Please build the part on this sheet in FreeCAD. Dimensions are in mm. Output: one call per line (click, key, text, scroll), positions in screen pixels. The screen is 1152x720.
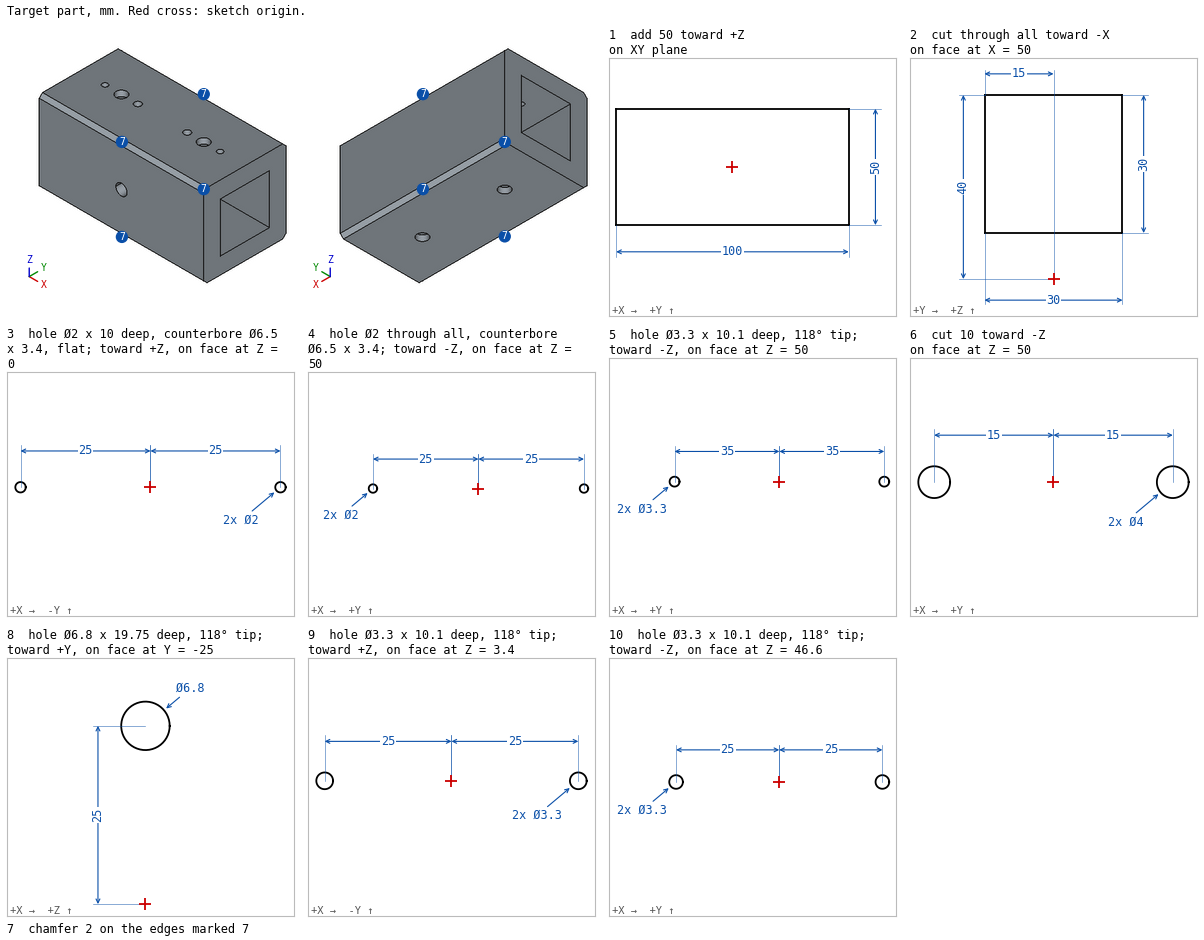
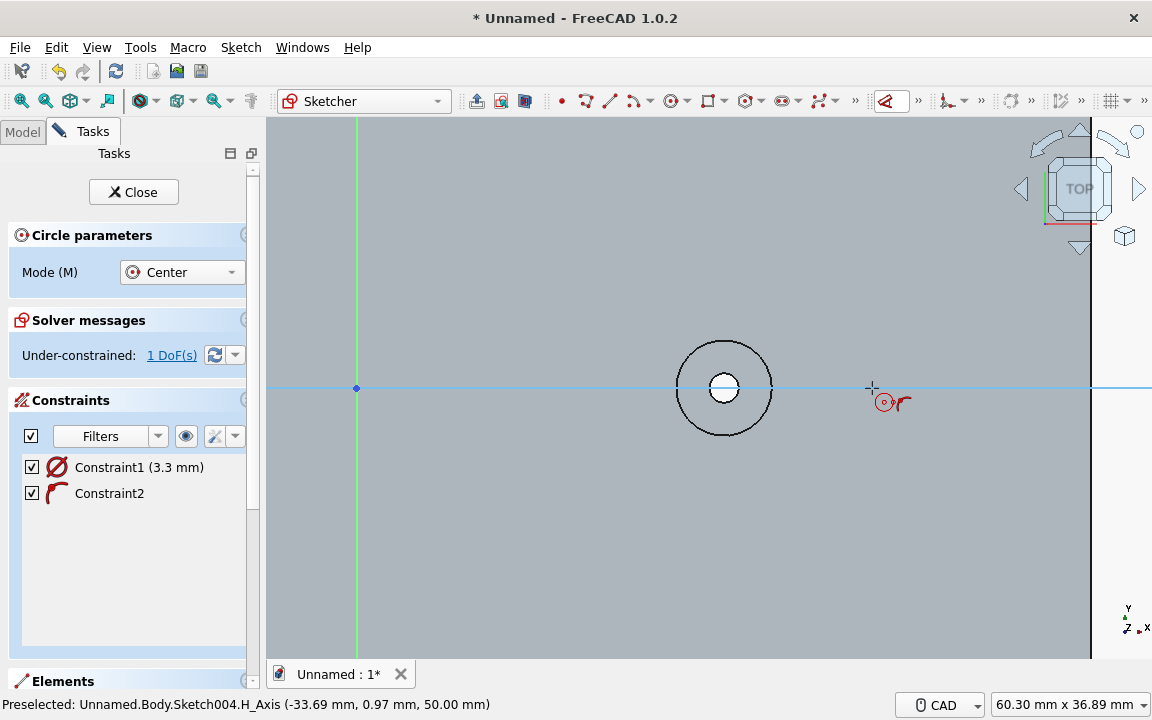
click(871, 388)
move(888, 371)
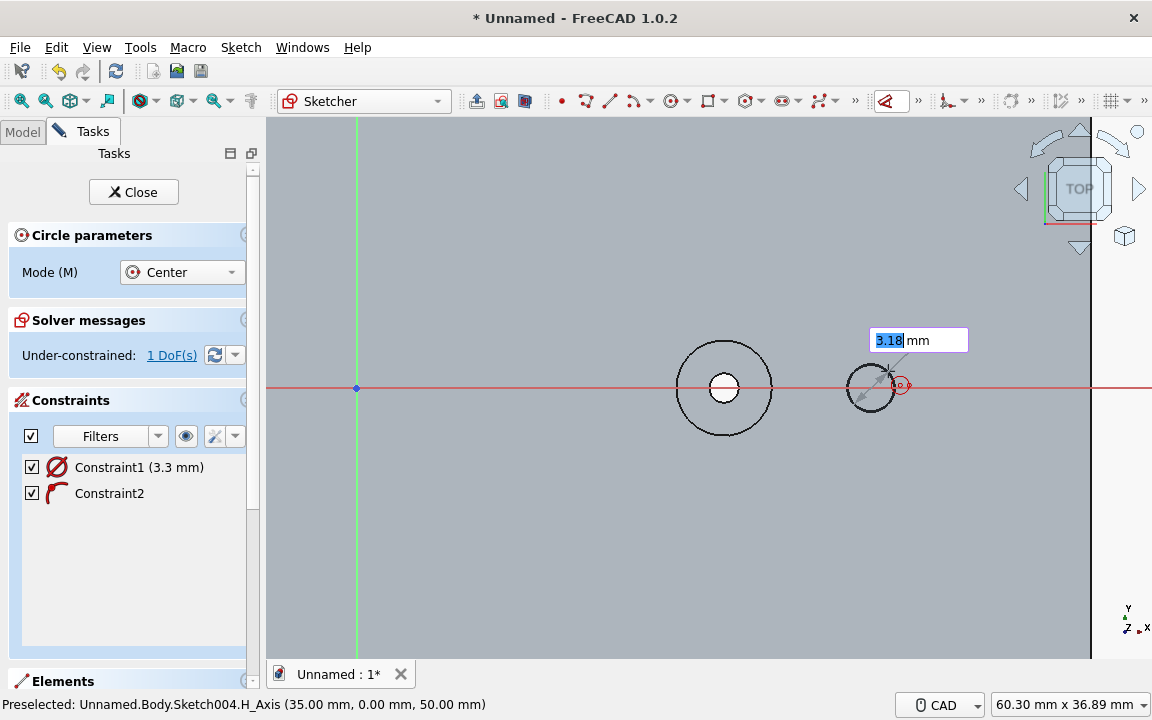
text(3.3)
key(Return)
key(Escape)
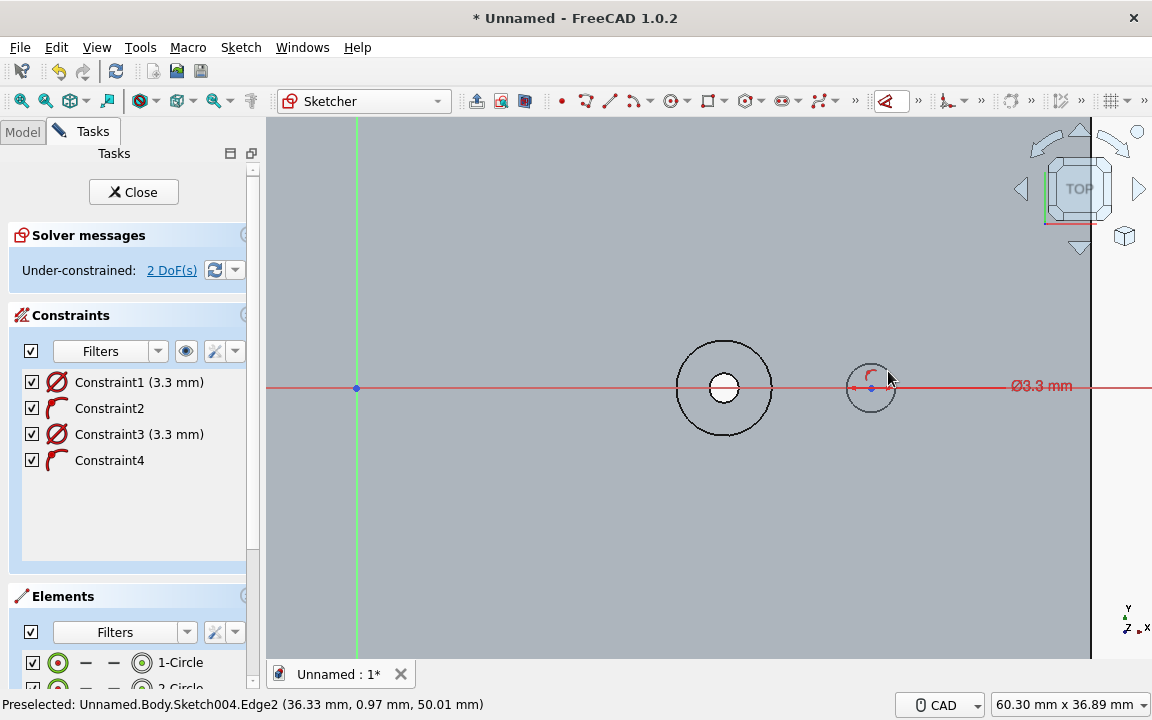
scroll(872, 388, down, 4)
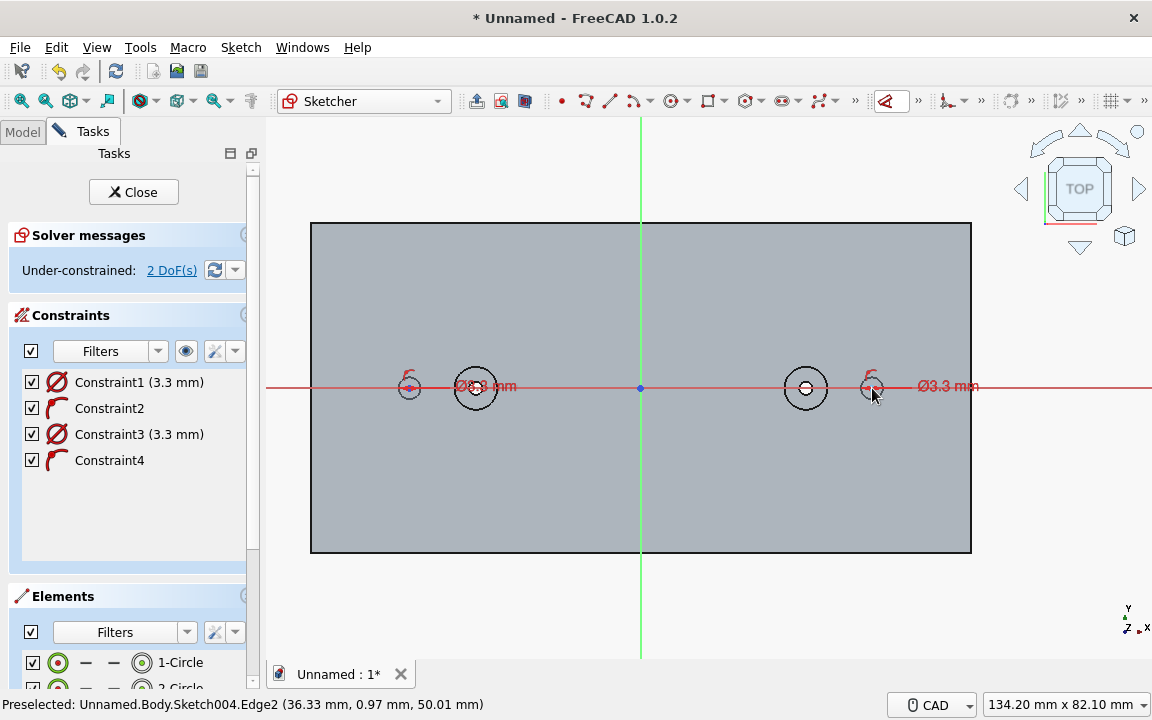
click(410, 388)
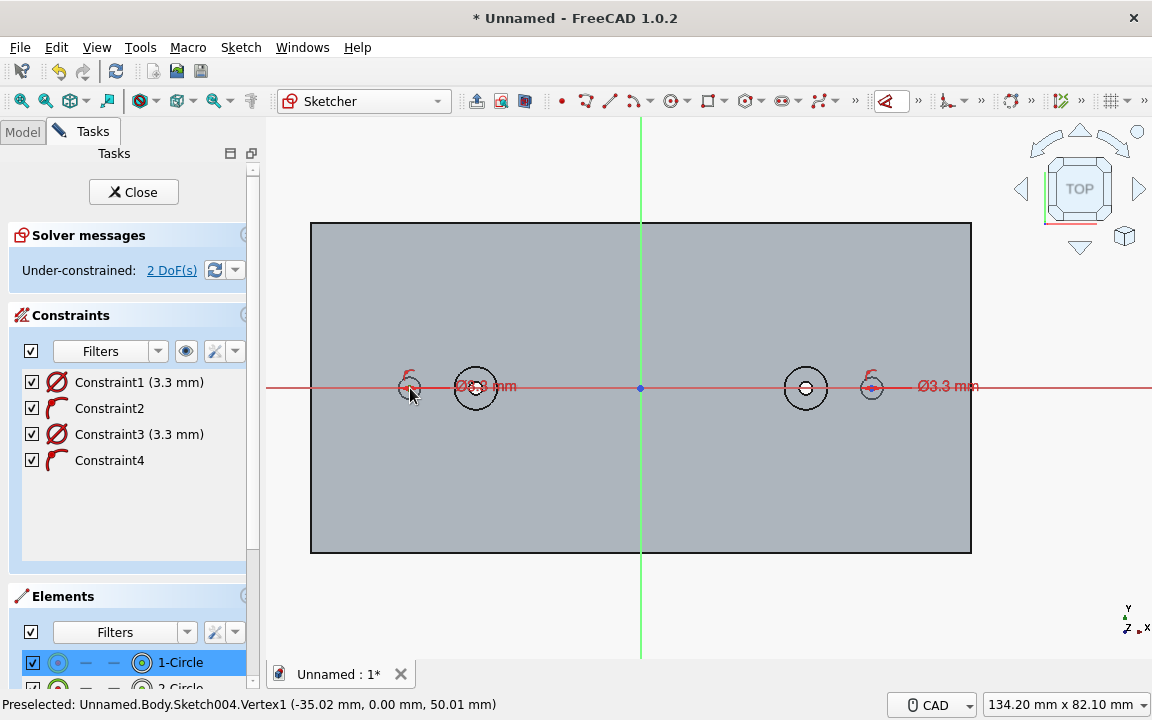
key(l)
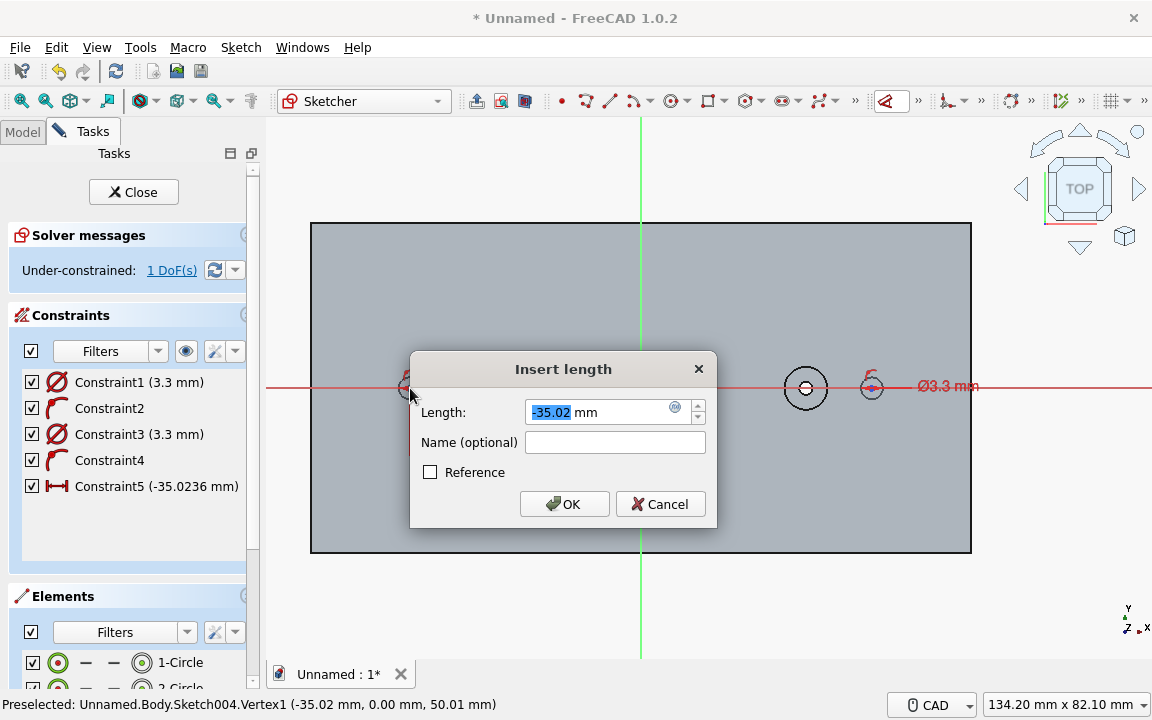
text(-35)
key(Return)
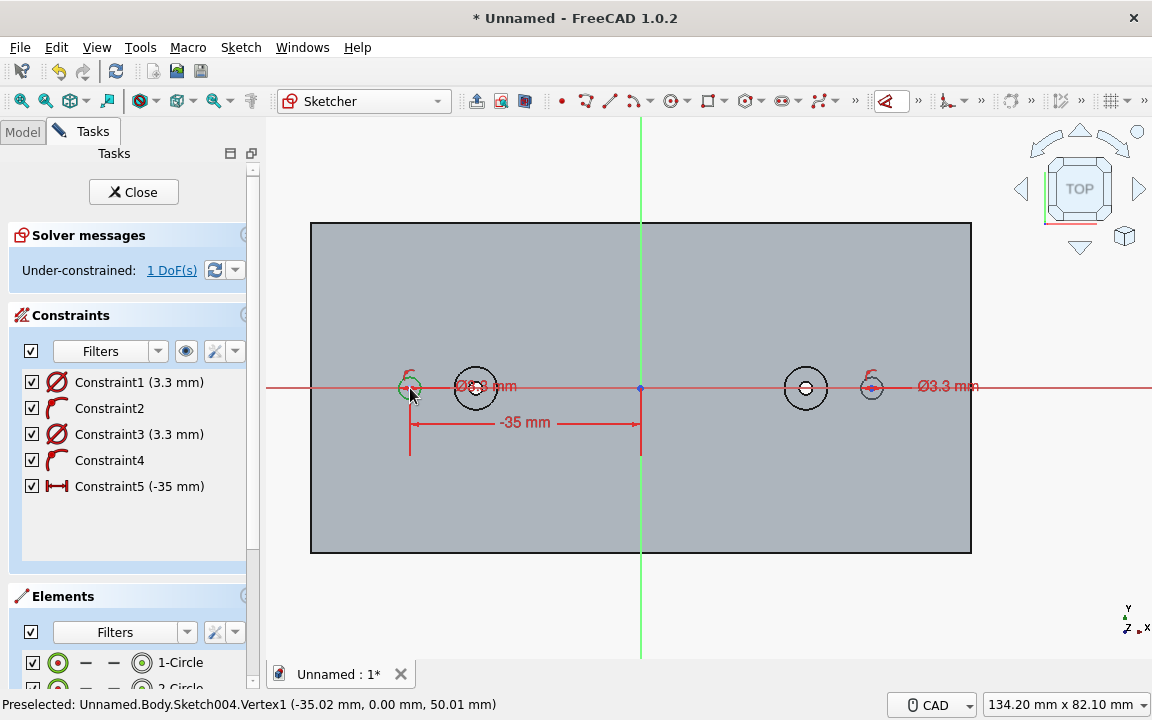
click(872, 388)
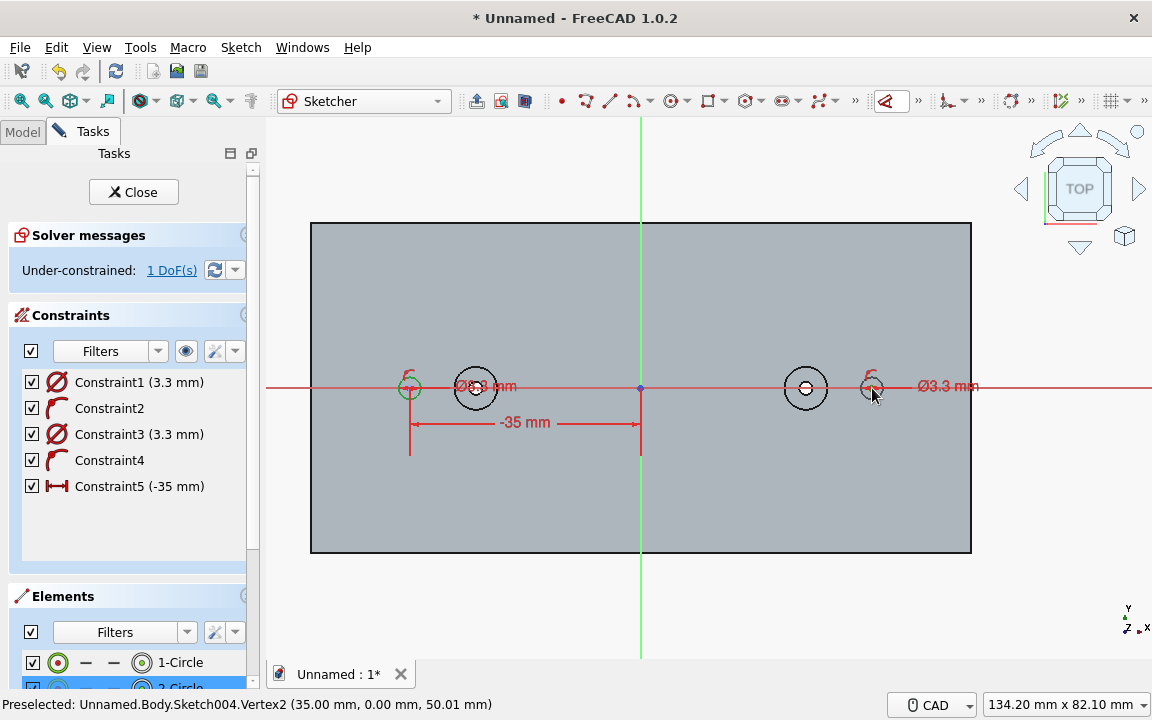
key(l)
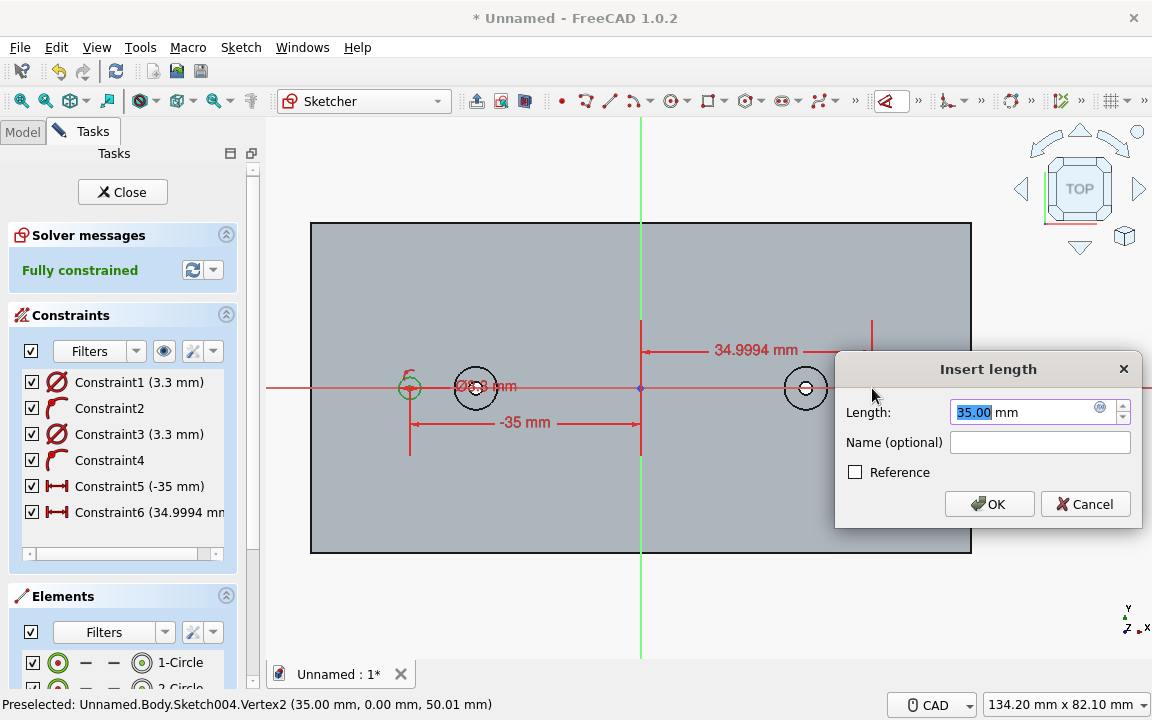
text(35)
key(Return)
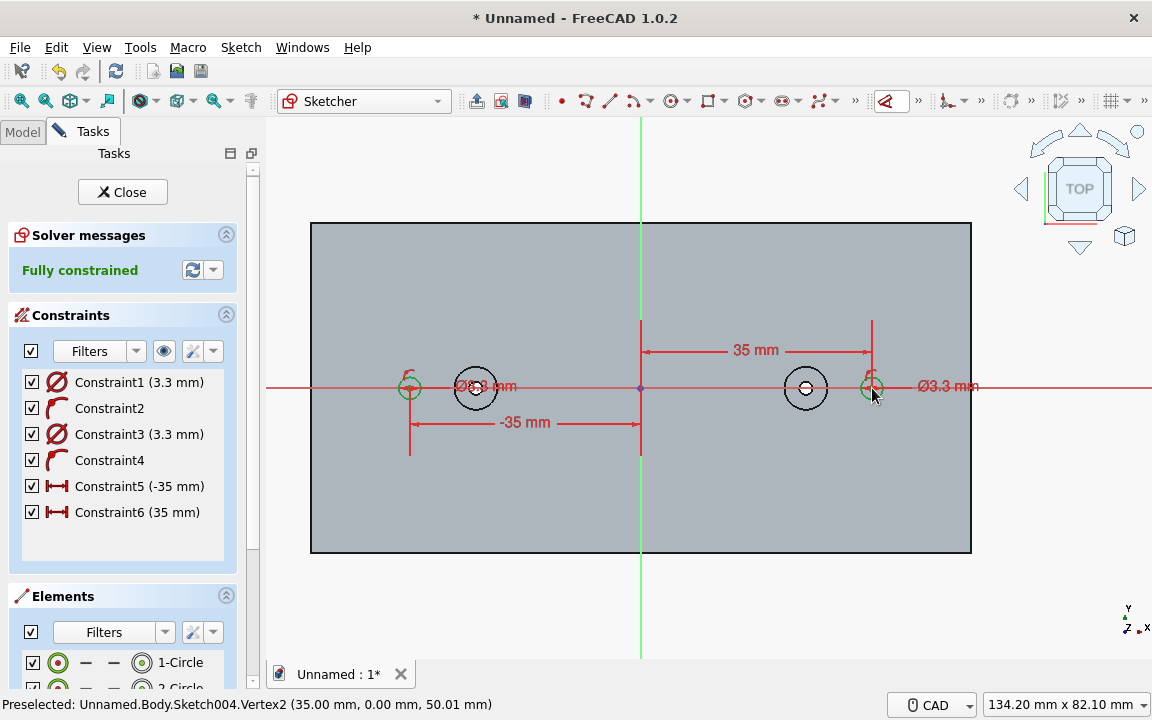
click(123, 192)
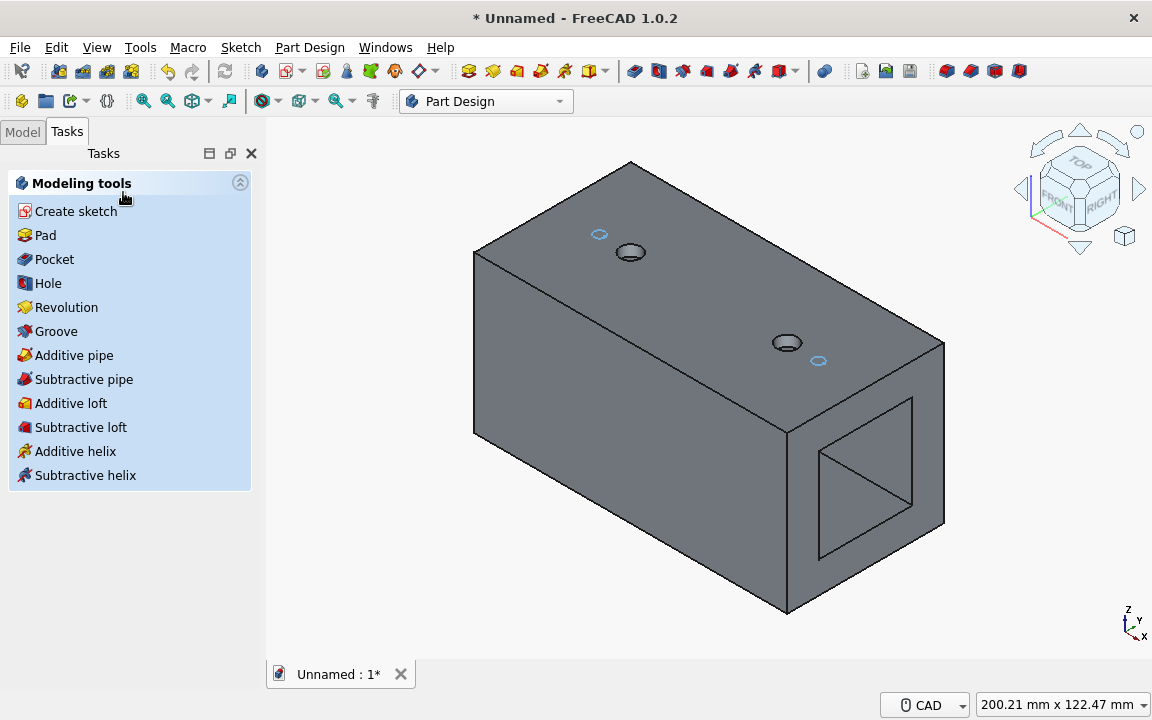
click(660, 72)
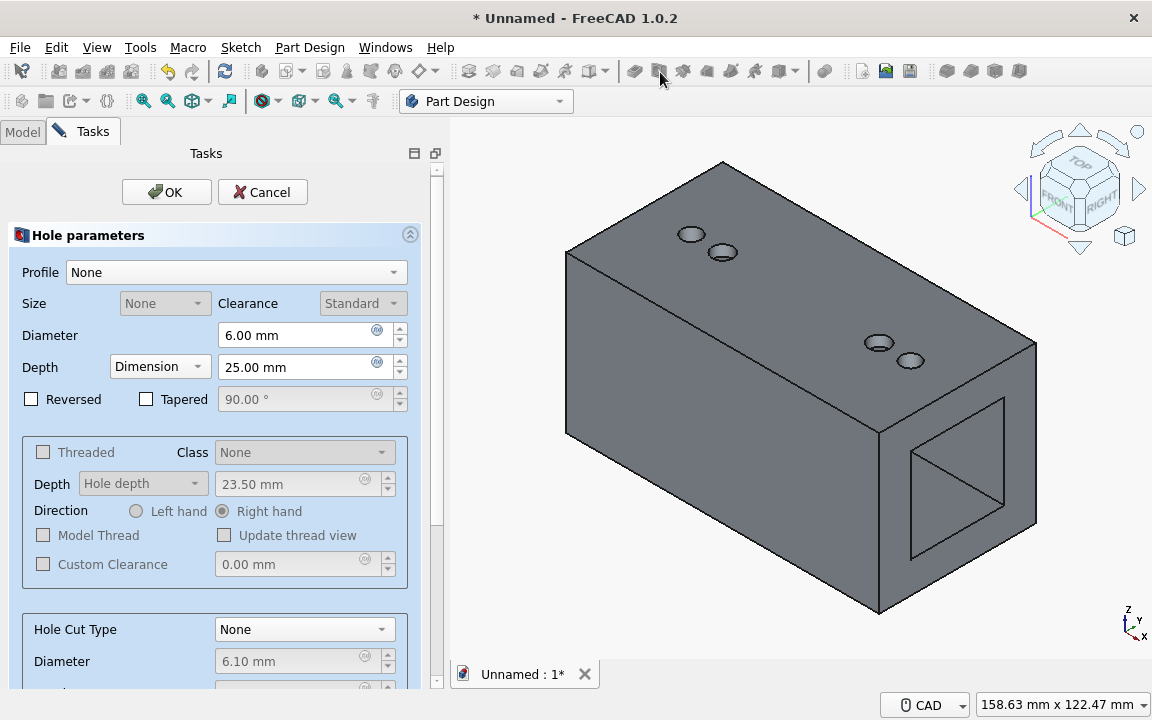
triple_click(305, 335)